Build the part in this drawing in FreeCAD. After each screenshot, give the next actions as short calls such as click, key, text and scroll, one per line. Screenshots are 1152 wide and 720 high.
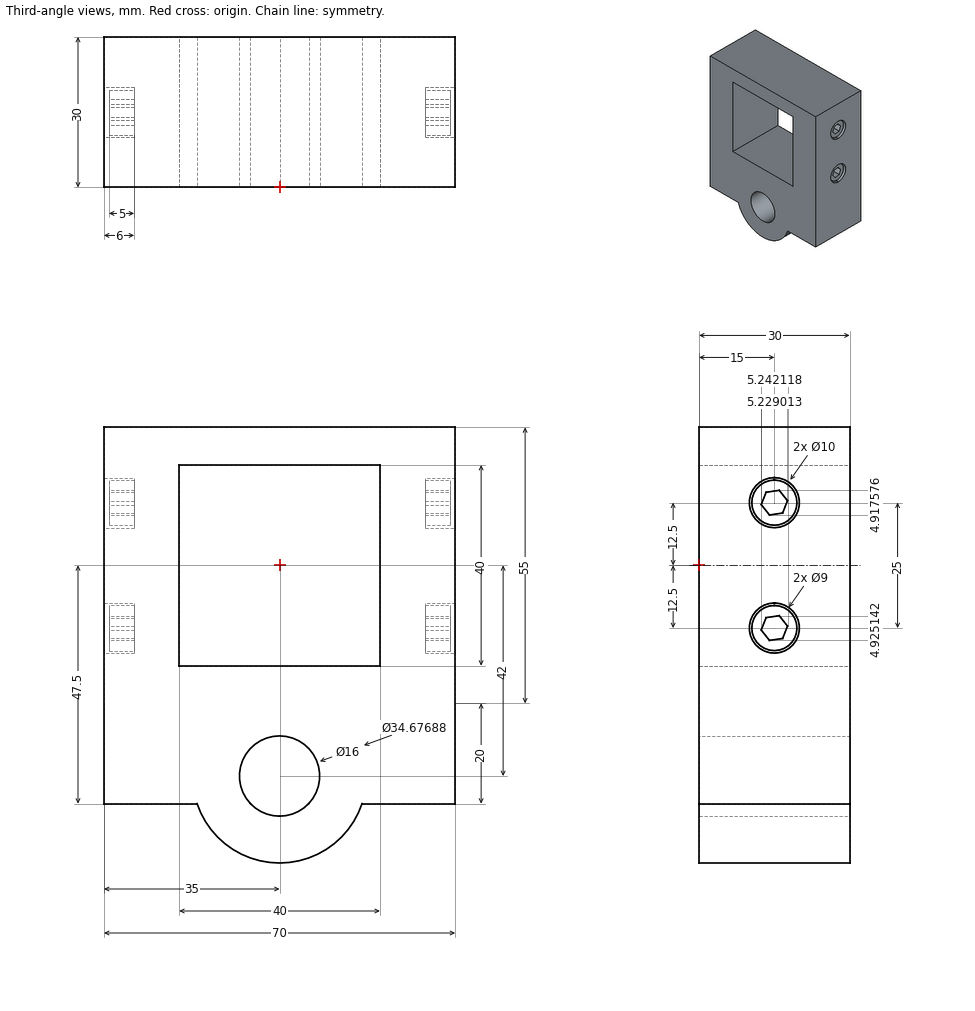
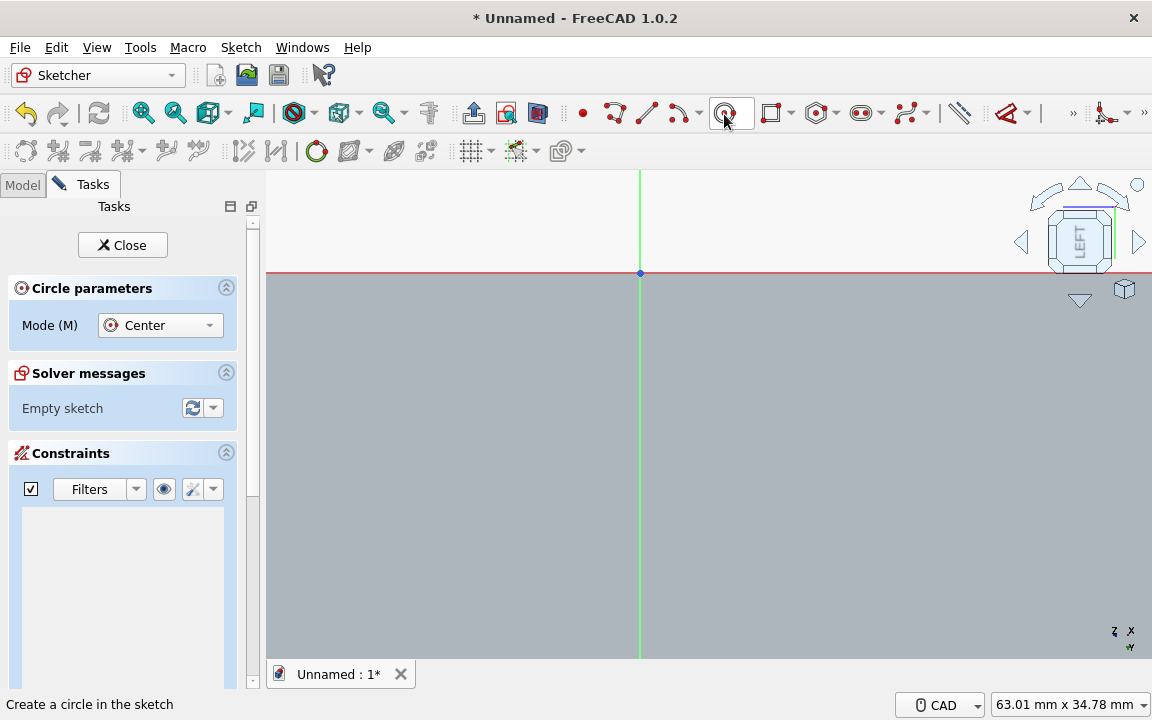
click(464, 484)
move(514, 435)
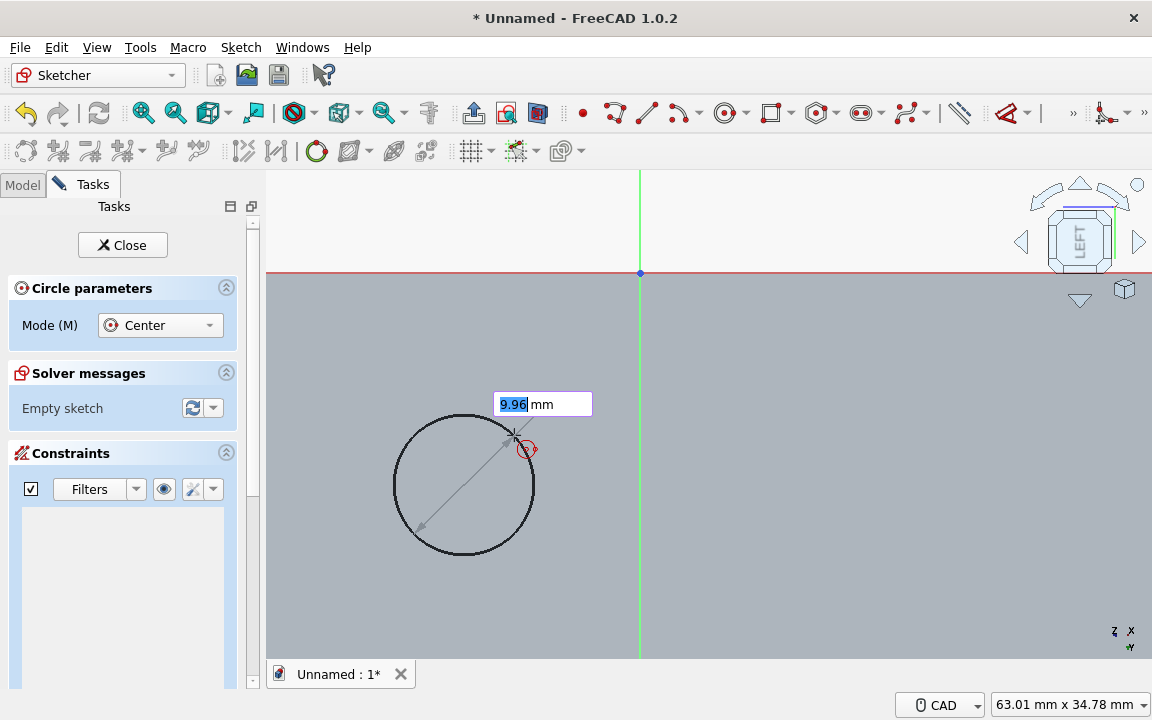
text(10)
key(Return)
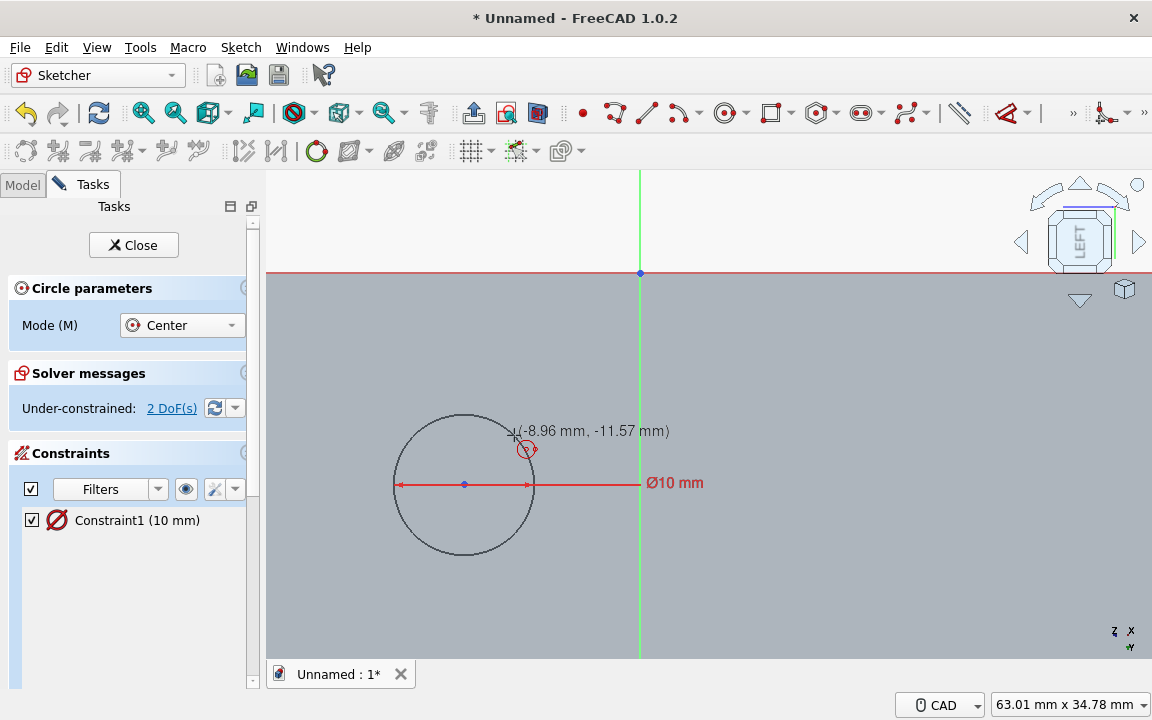
click(816, 484)
move(866, 435)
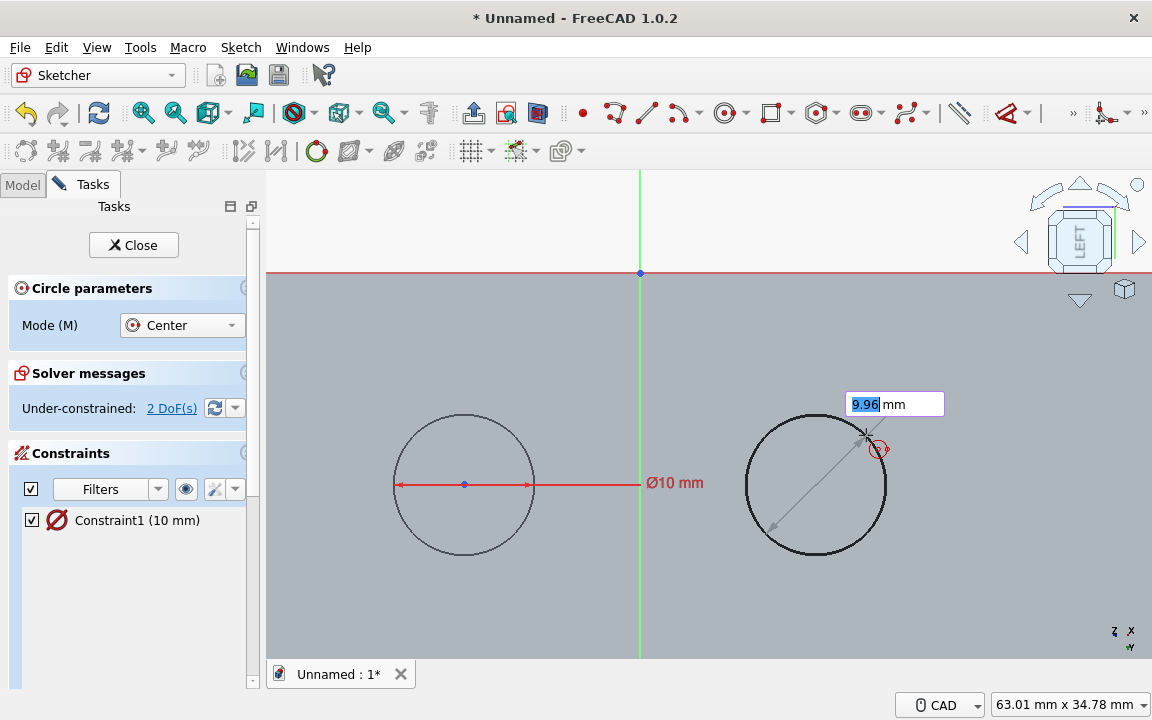
text(10)
key(Return)
key(Escape)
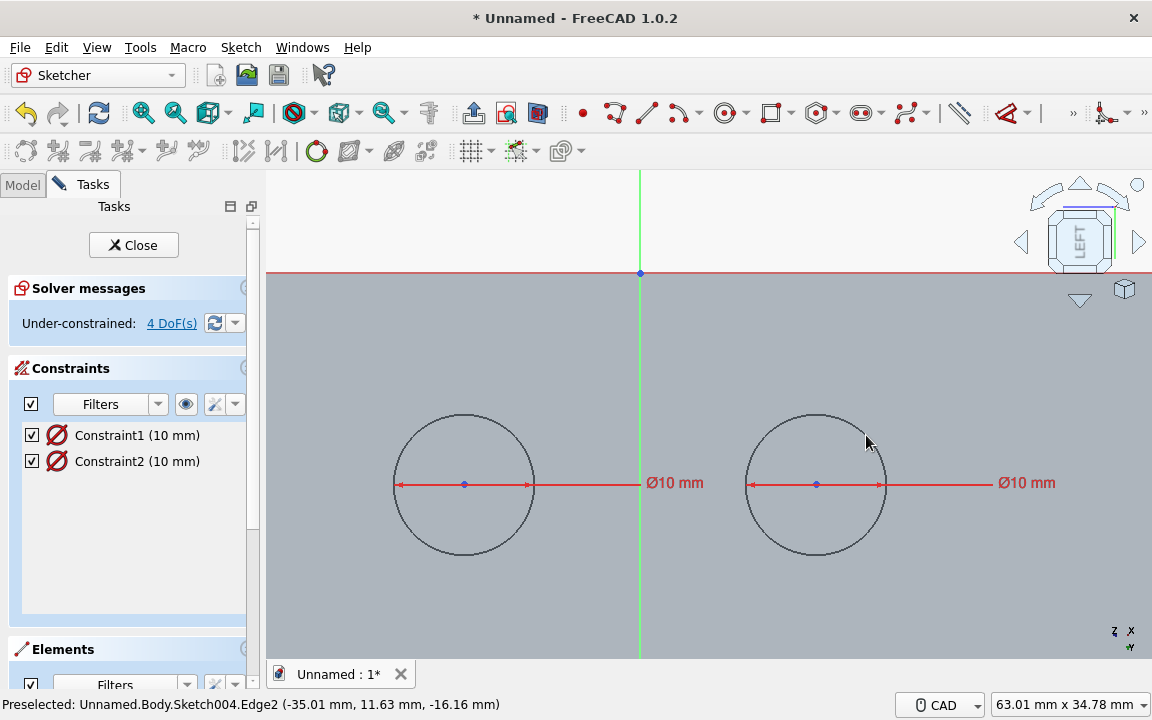
click(464, 485)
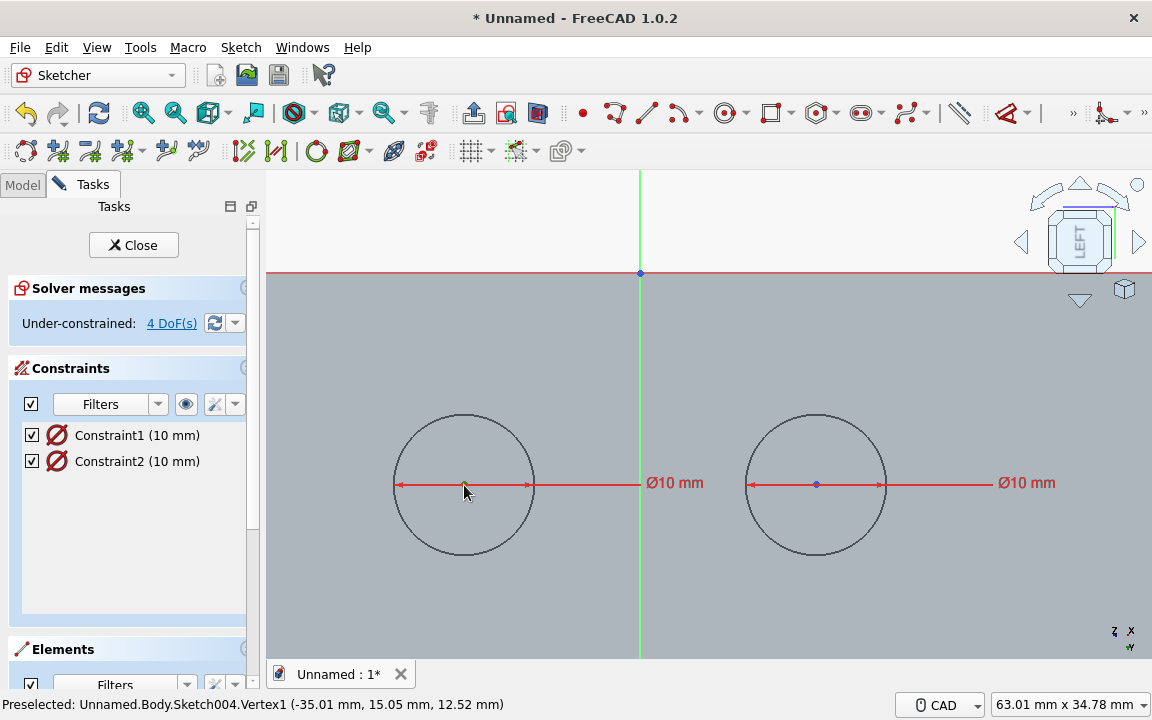
click(816, 485)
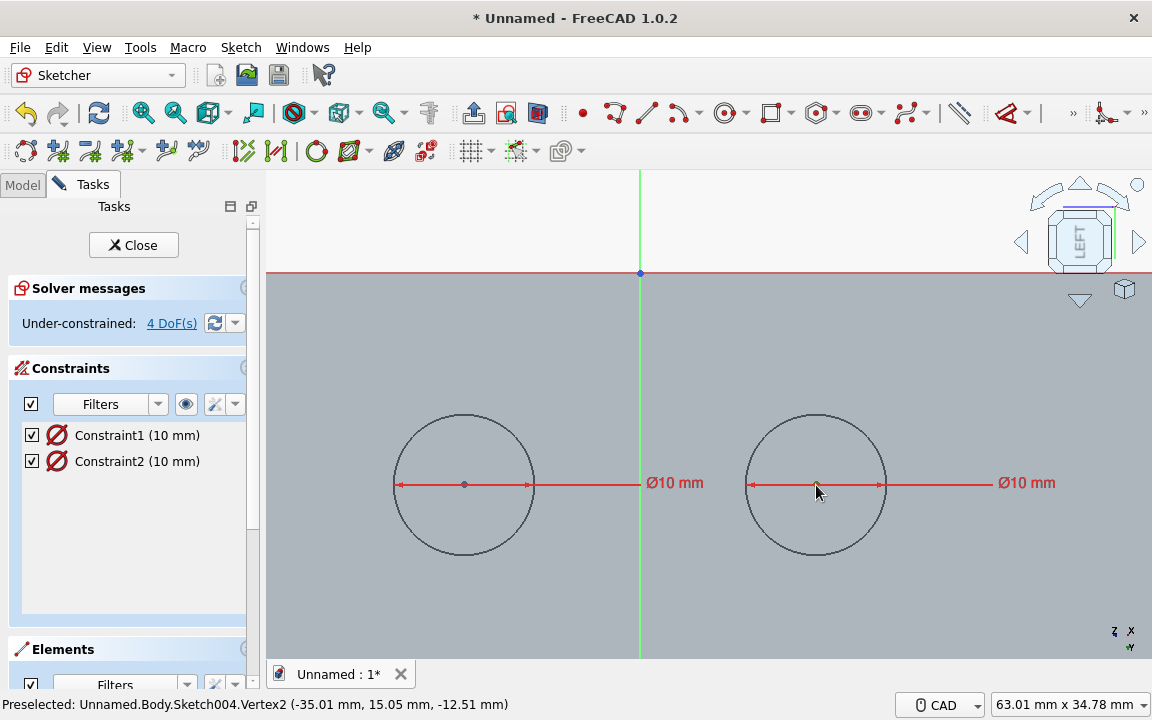
key(h)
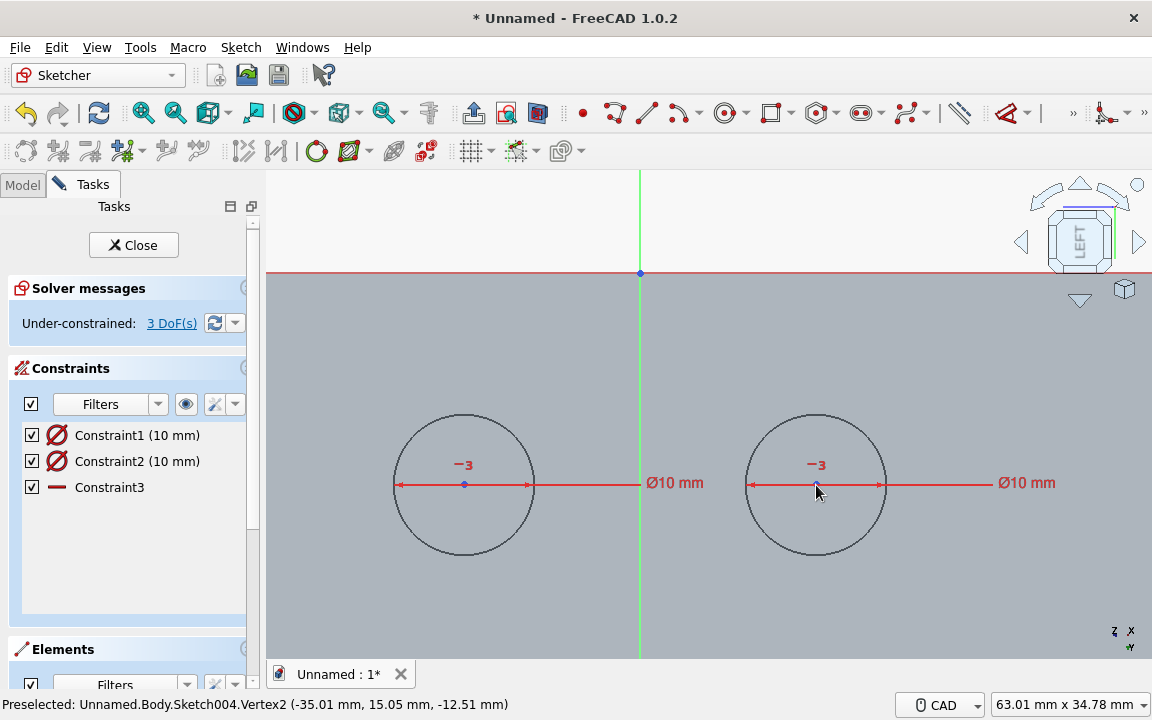
click(1006, 114)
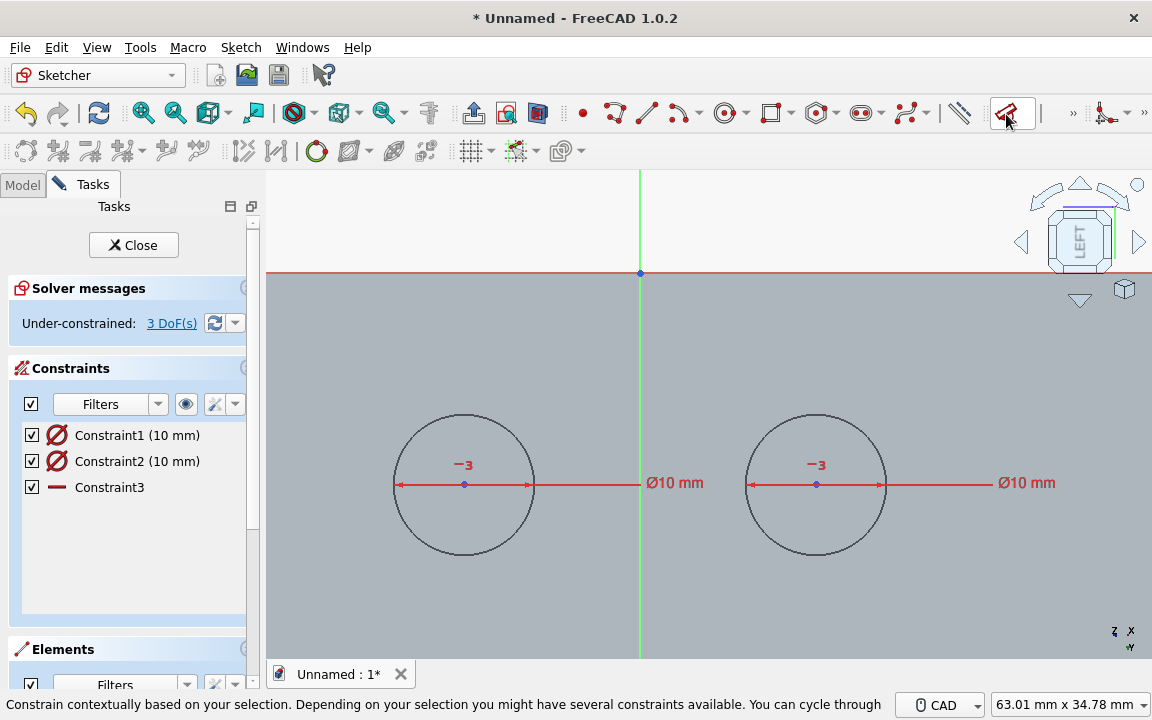
click(464, 485)
click(430, 379)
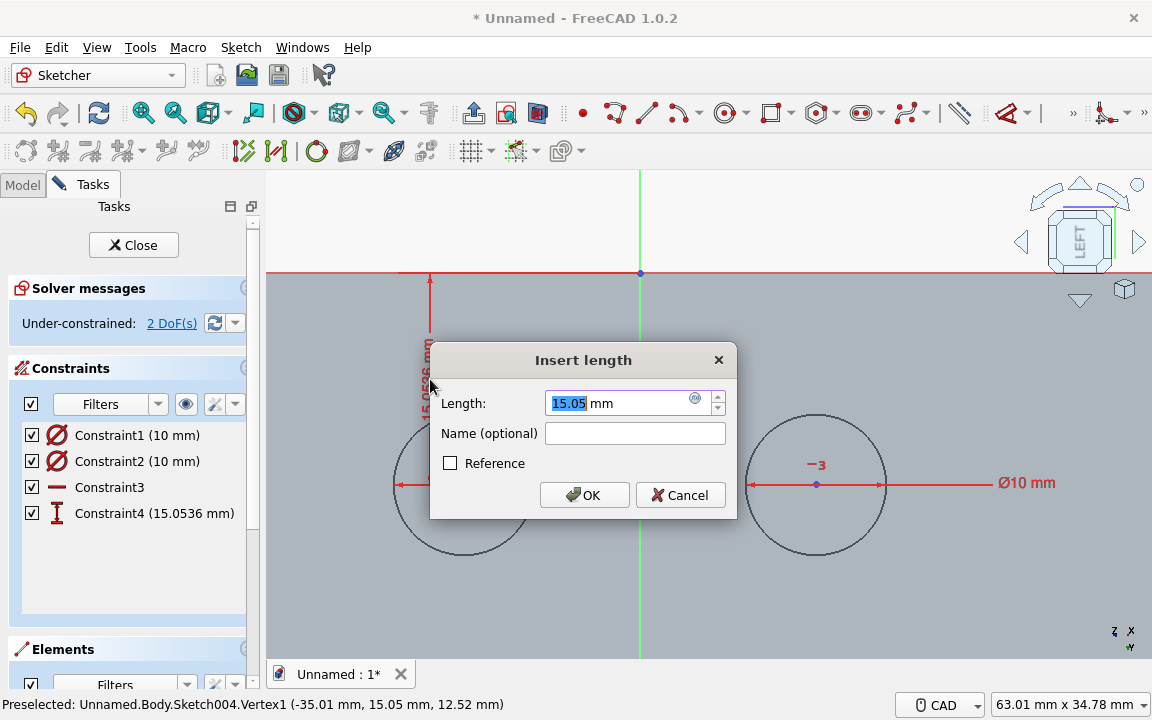
text(15)
key(Return)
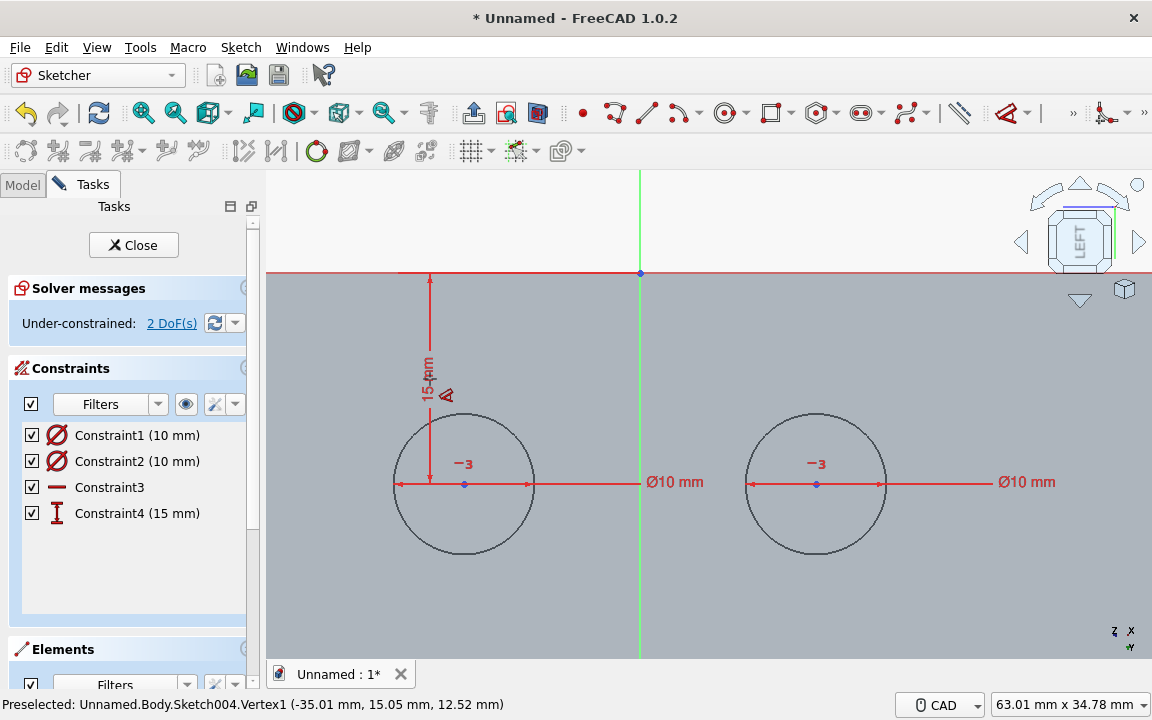
click(464, 484)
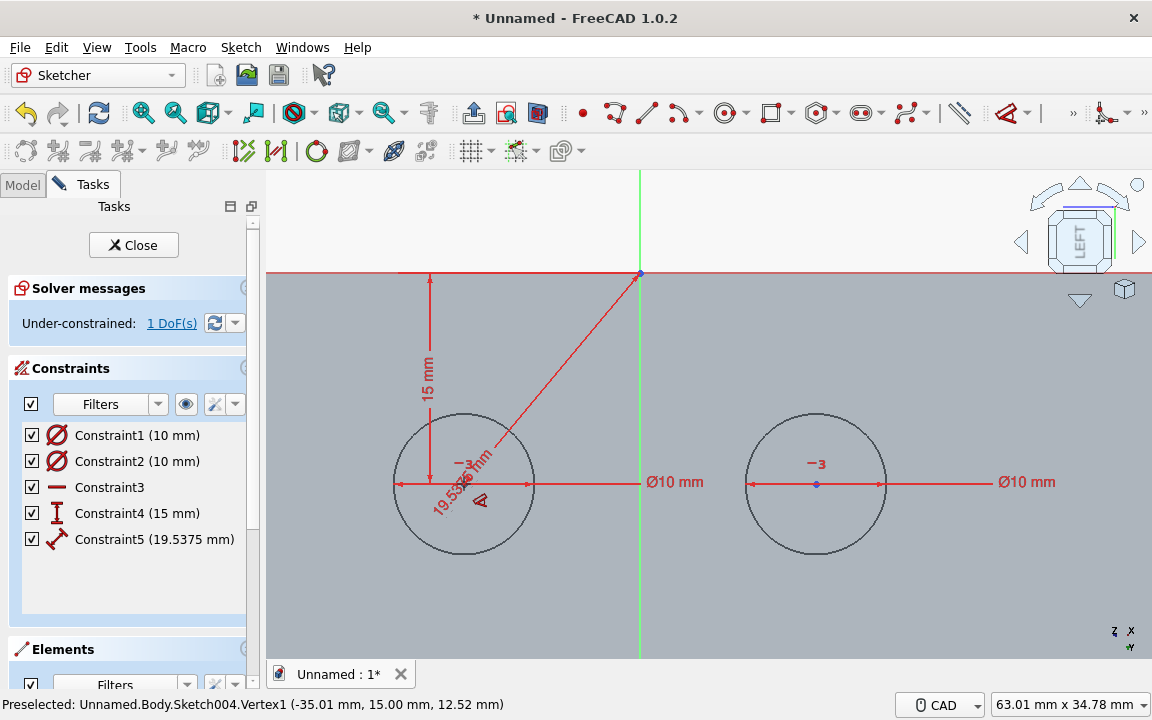
click(816, 484)
click(559, 518)